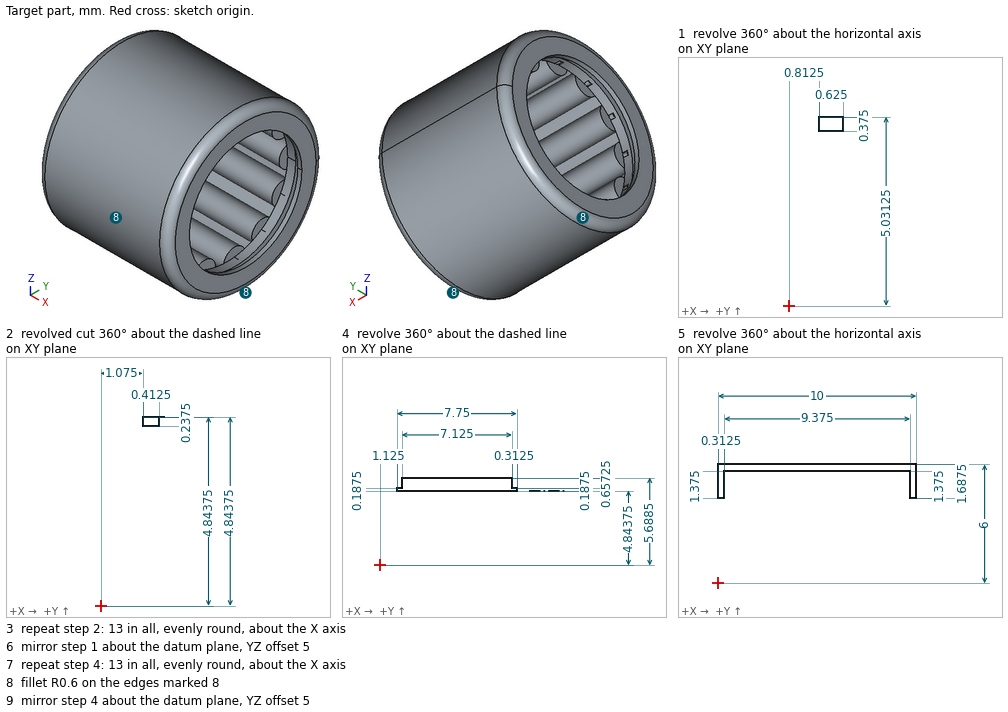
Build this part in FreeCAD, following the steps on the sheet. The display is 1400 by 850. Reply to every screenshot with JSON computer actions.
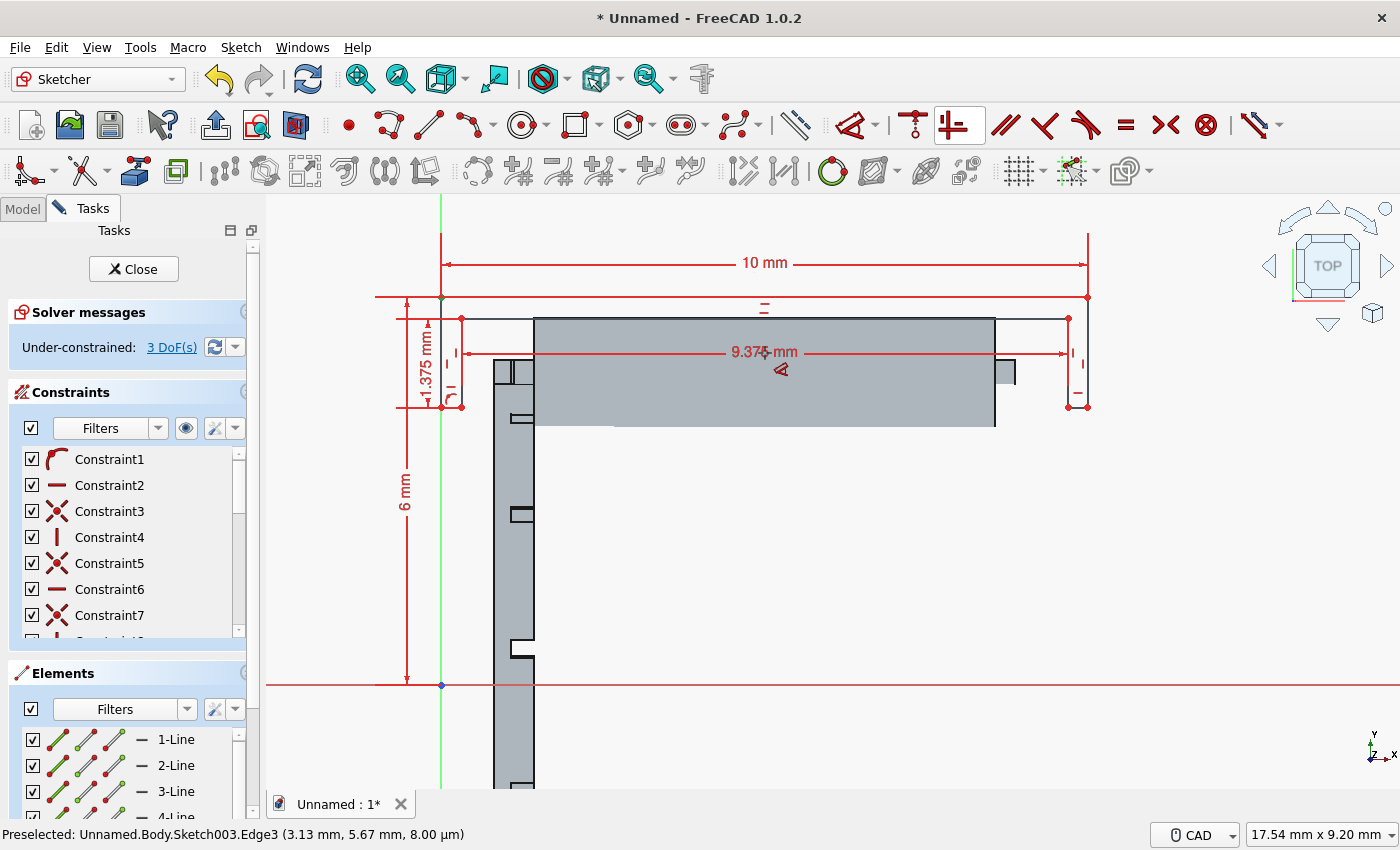
{"action": "left_click", "coordinate": [1068, 345]}
{"action": "left_click", "coordinate": [1102, 363]}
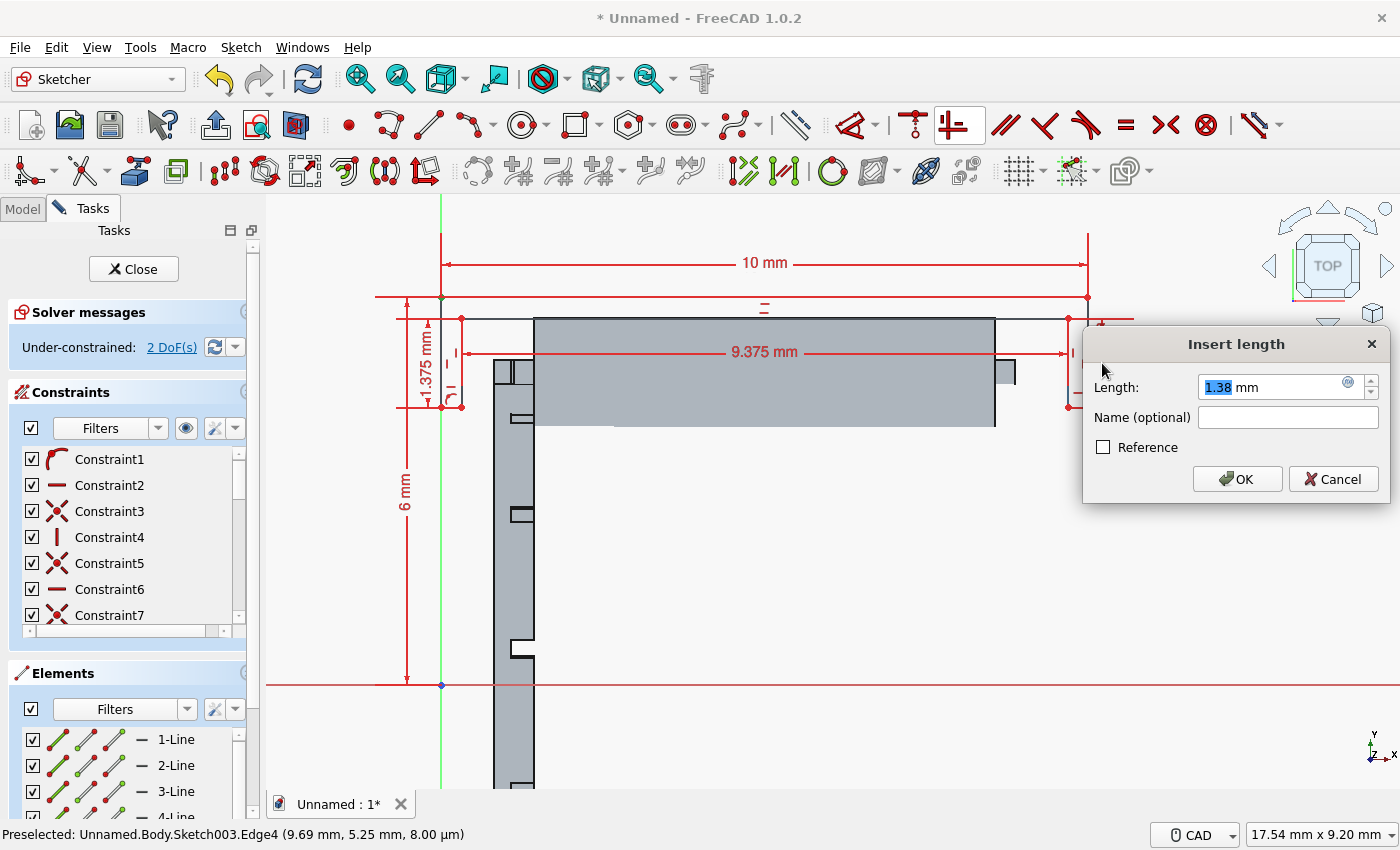
{"action": "type", "text": "1.375"}
{"action": "key", "text": "Return"}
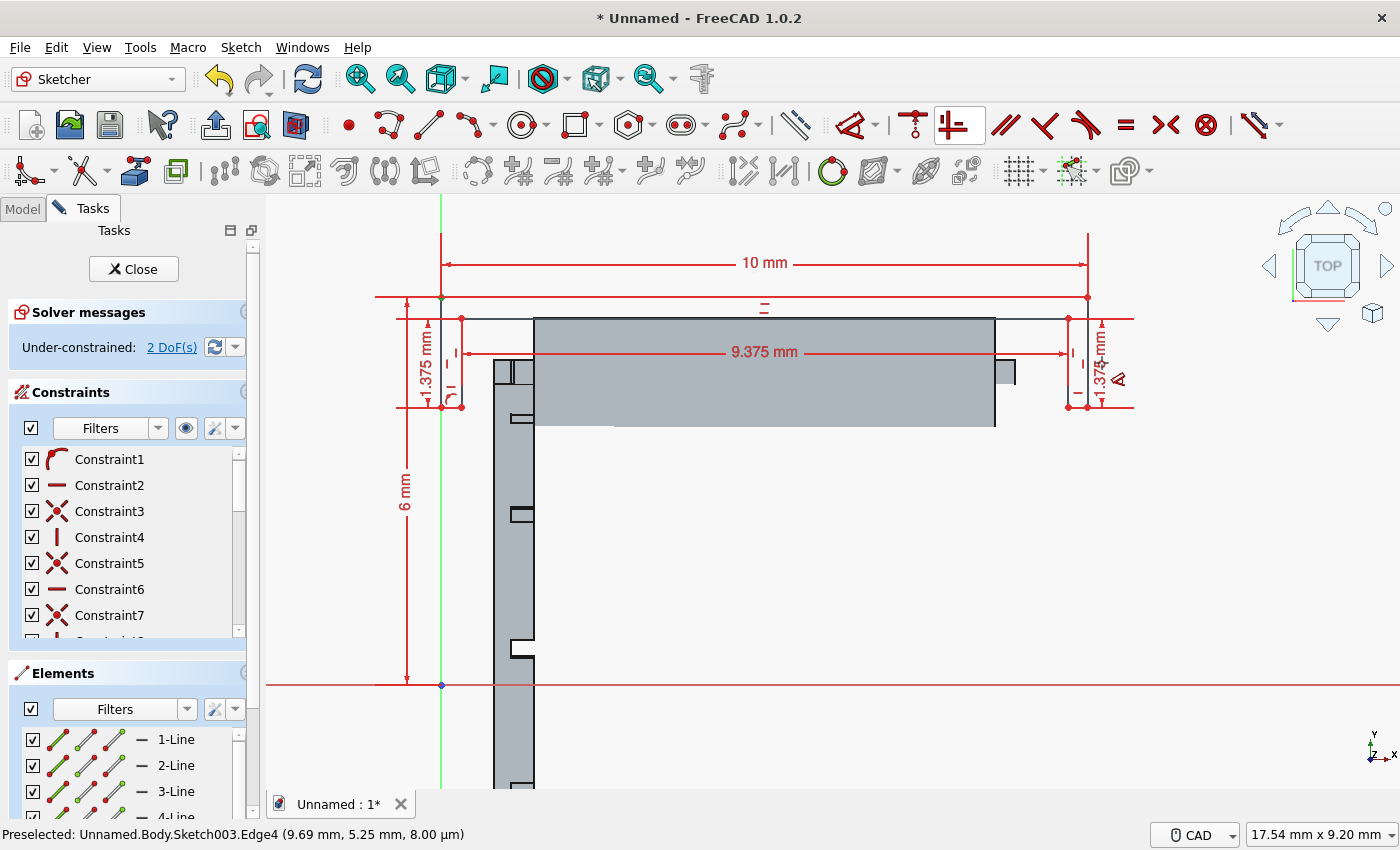
{"action": "scroll", "coordinate": [452, 408], "scroll_direction": "up", "scroll_amount": 4}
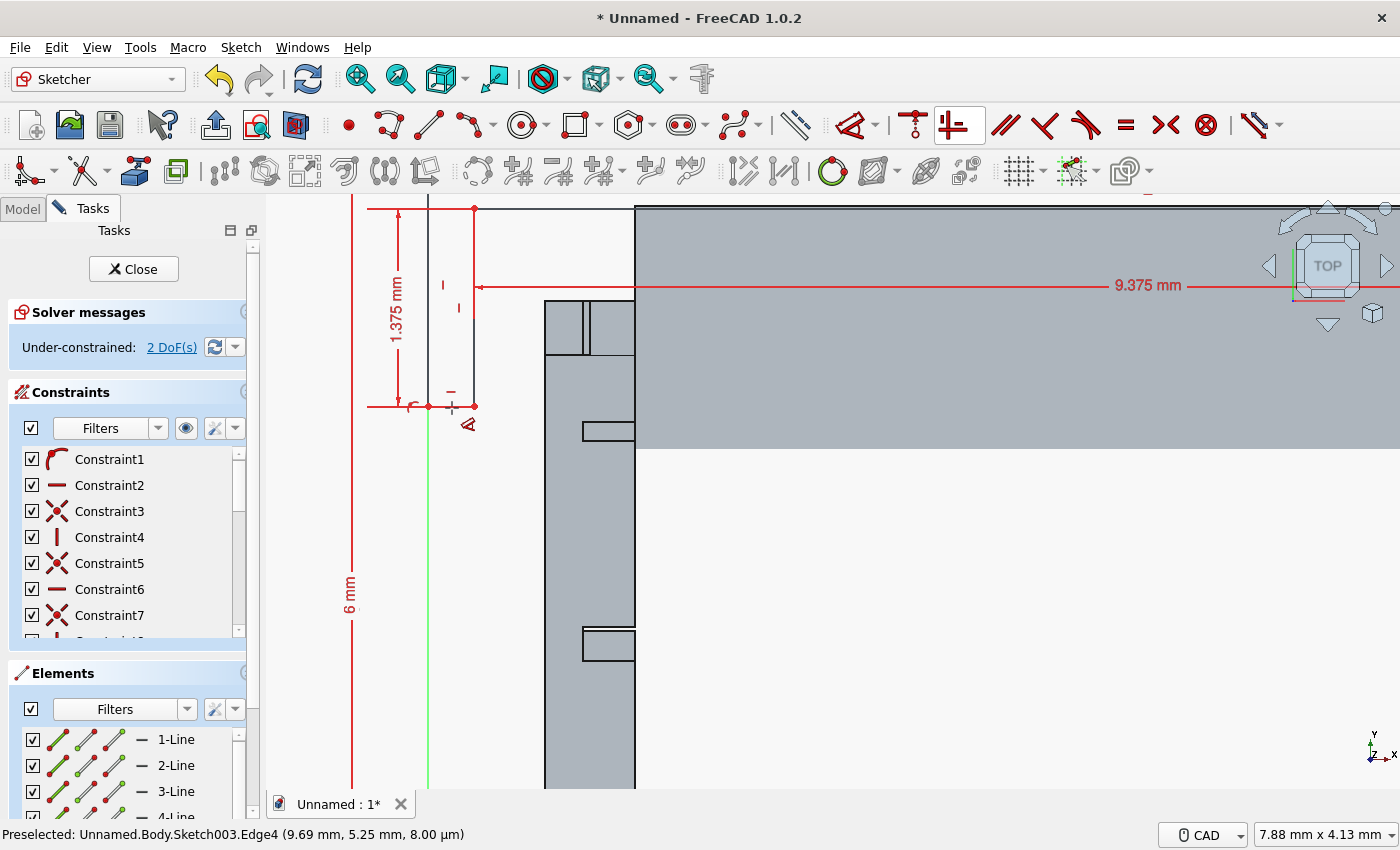
{"action": "left_click", "coordinate": [451, 407]}
{"action": "left_click", "coordinate": [451, 373]}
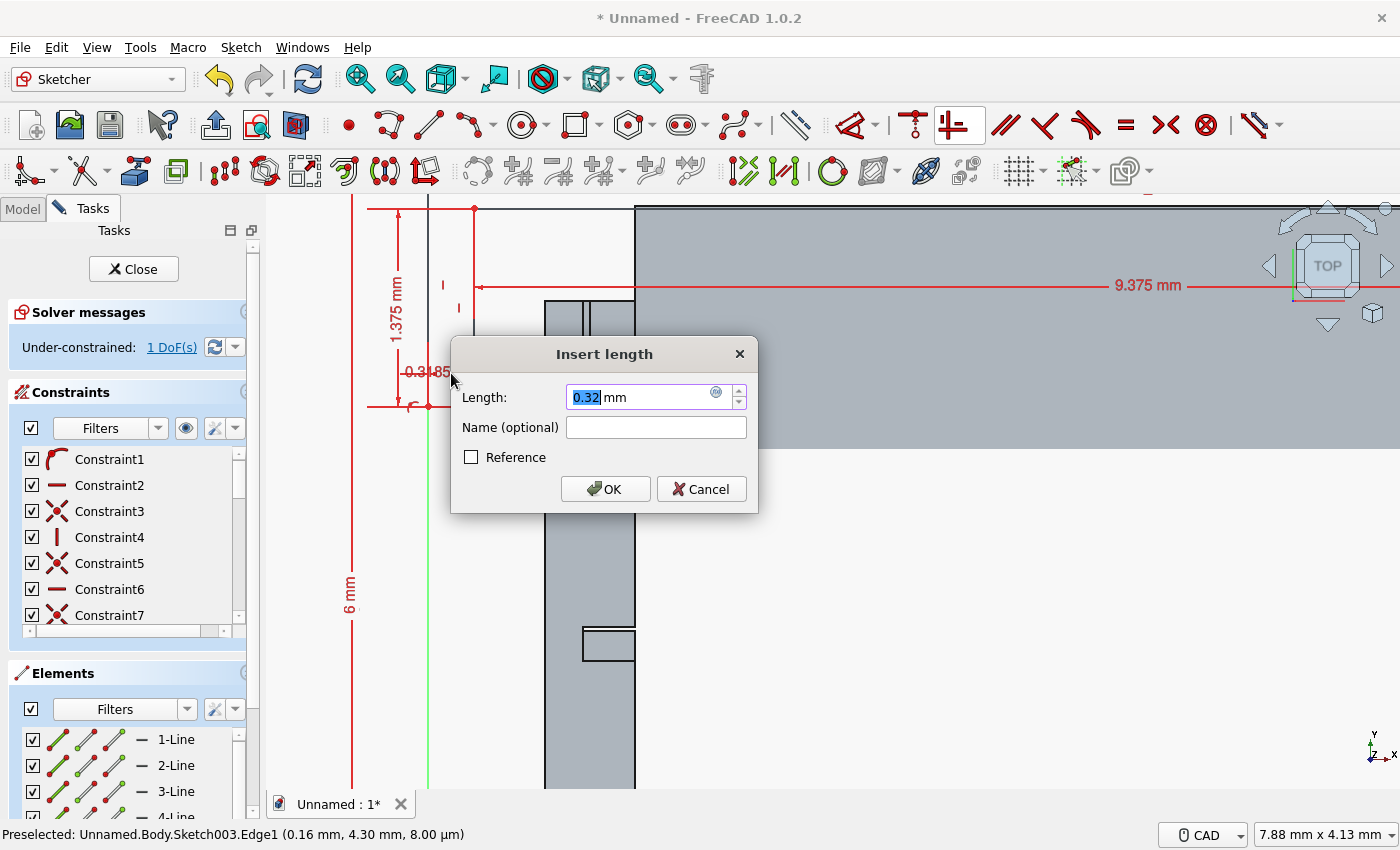
{"action": "type", "text": "0.3125"}
{"action": "key", "text": "Return"}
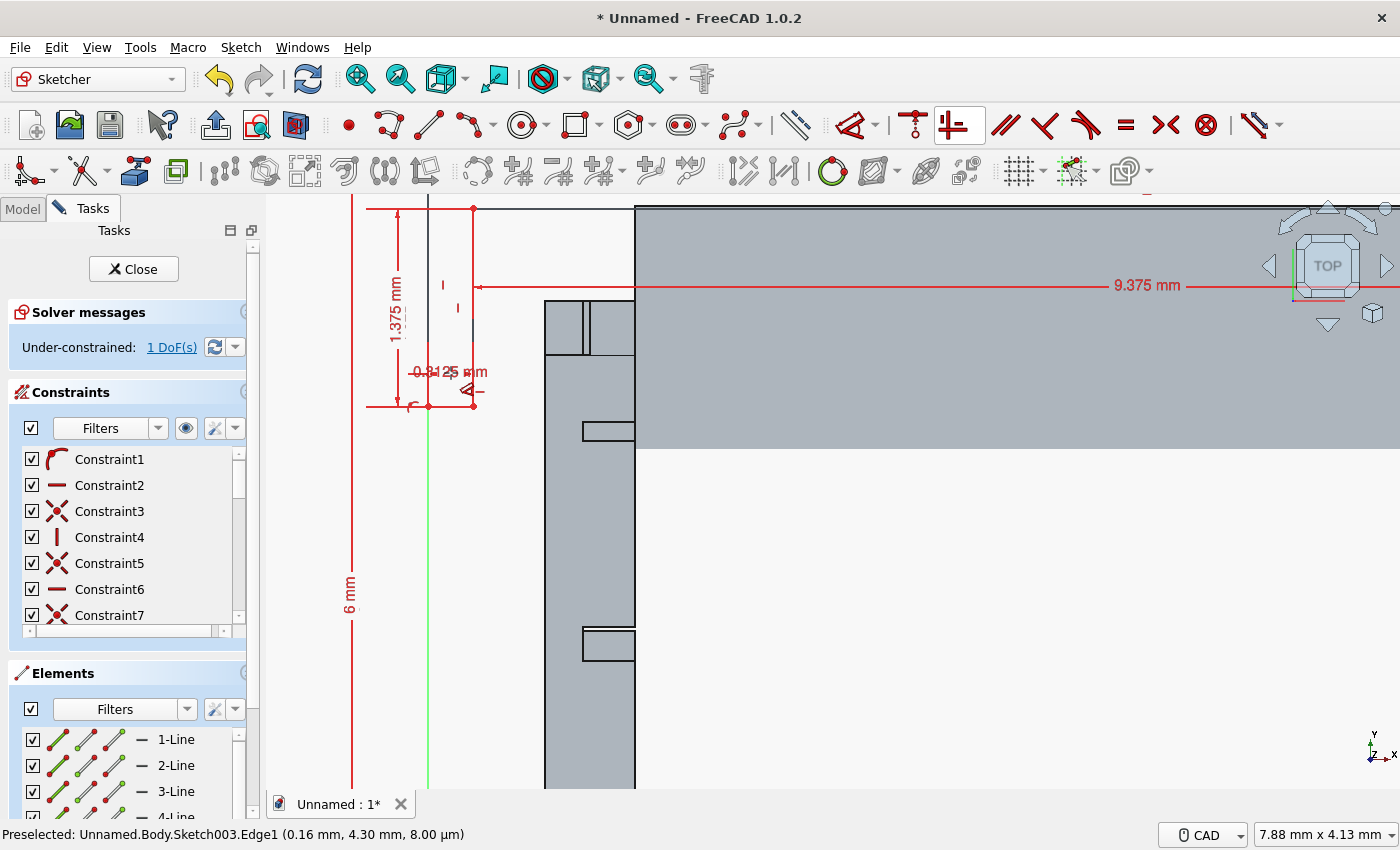
{"action": "scroll", "coordinate": [452, 409], "scroll_direction": "down", "scroll_amount": 4}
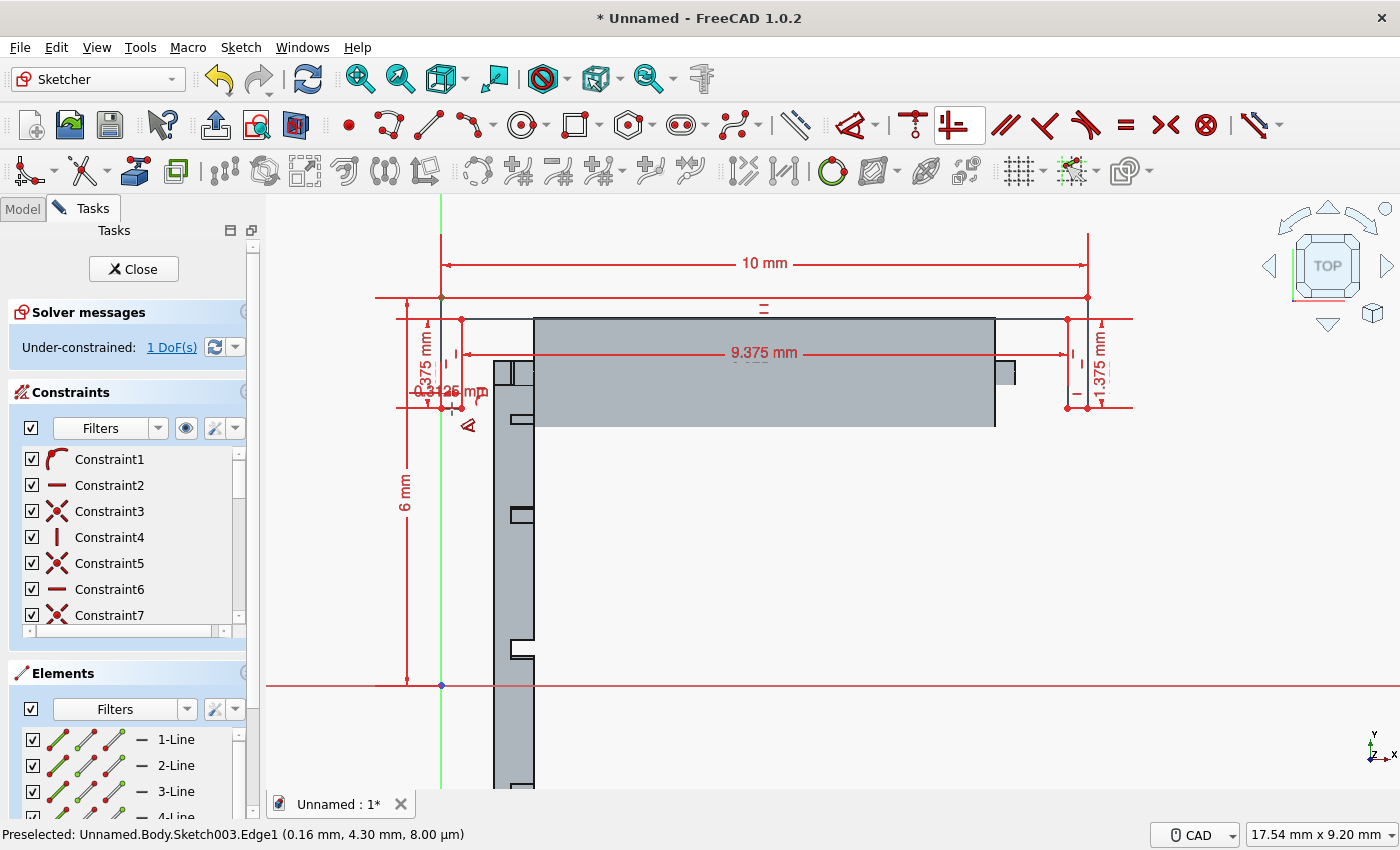
{"action": "left_click", "coordinate": [1088, 375]}
{"action": "left_click", "coordinate": [1122, 328]}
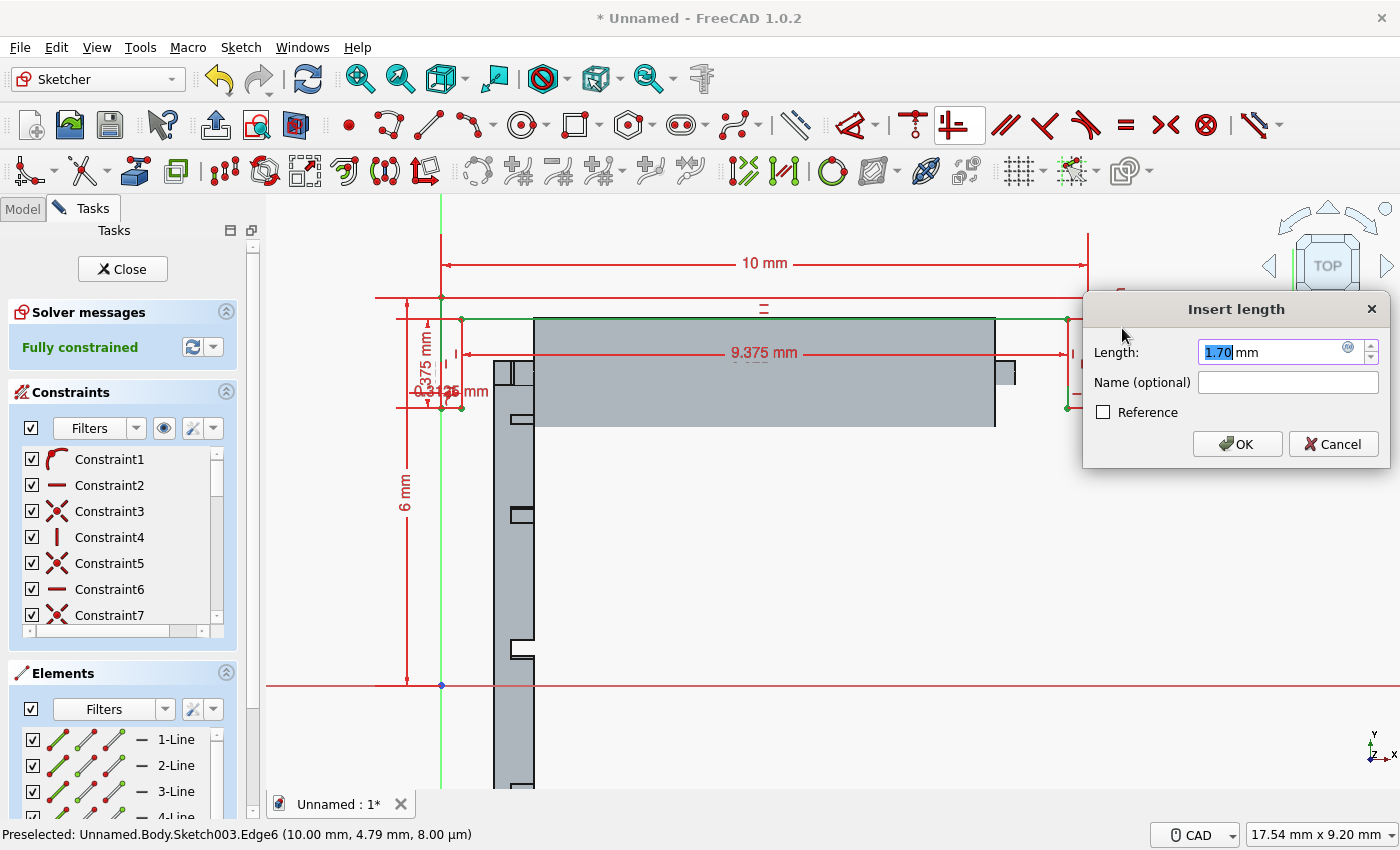
{"action": "type", "text": "1.6875"}
{"action": "key", "text": "Return"}
{"action": "key", "text": "Escape"}